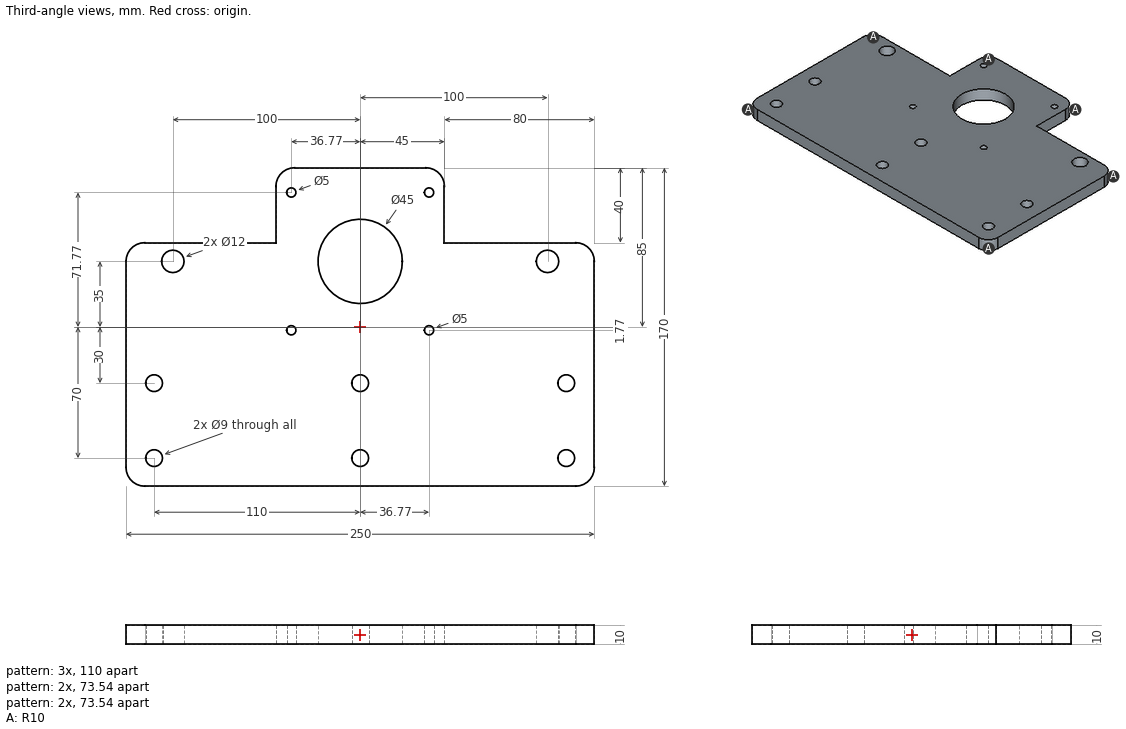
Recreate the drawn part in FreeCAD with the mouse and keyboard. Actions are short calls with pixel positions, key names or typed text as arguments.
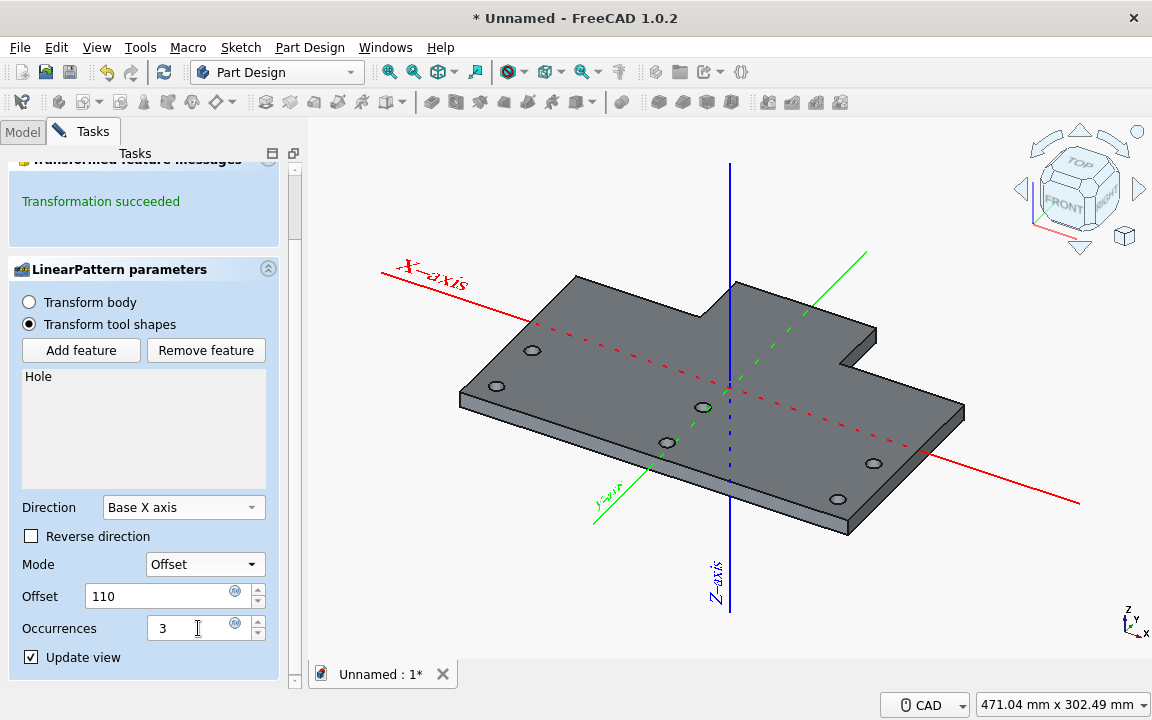
scroll(295, 426, up, 3)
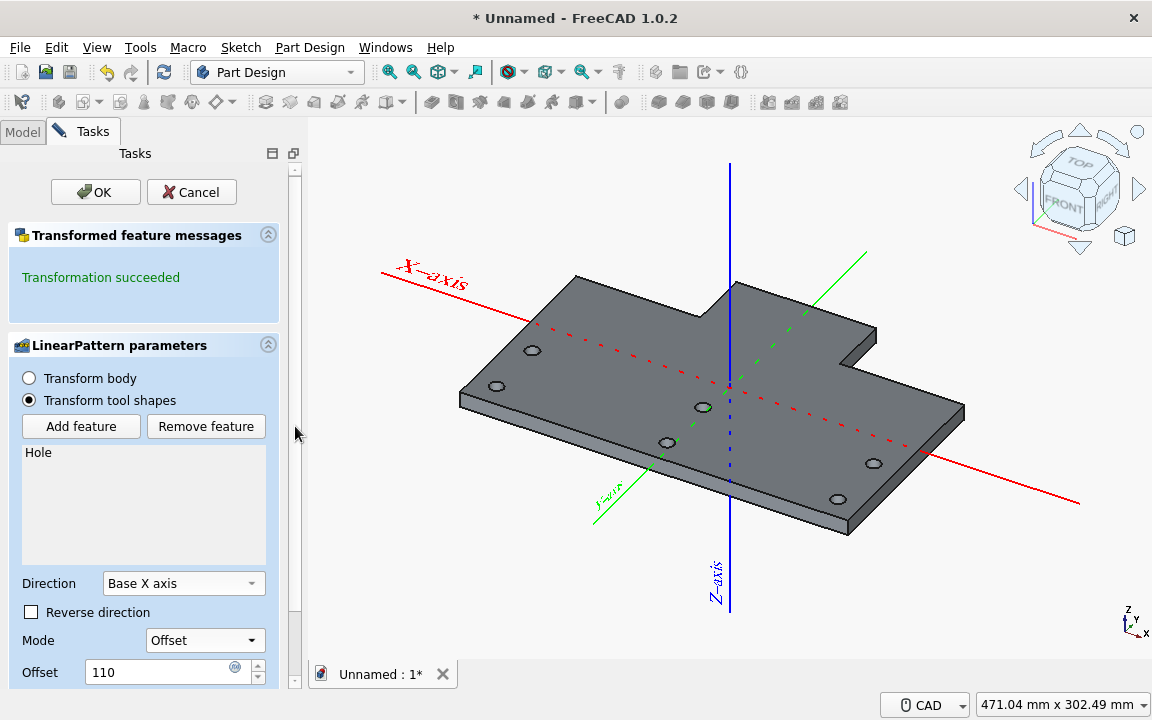
click(96, 192)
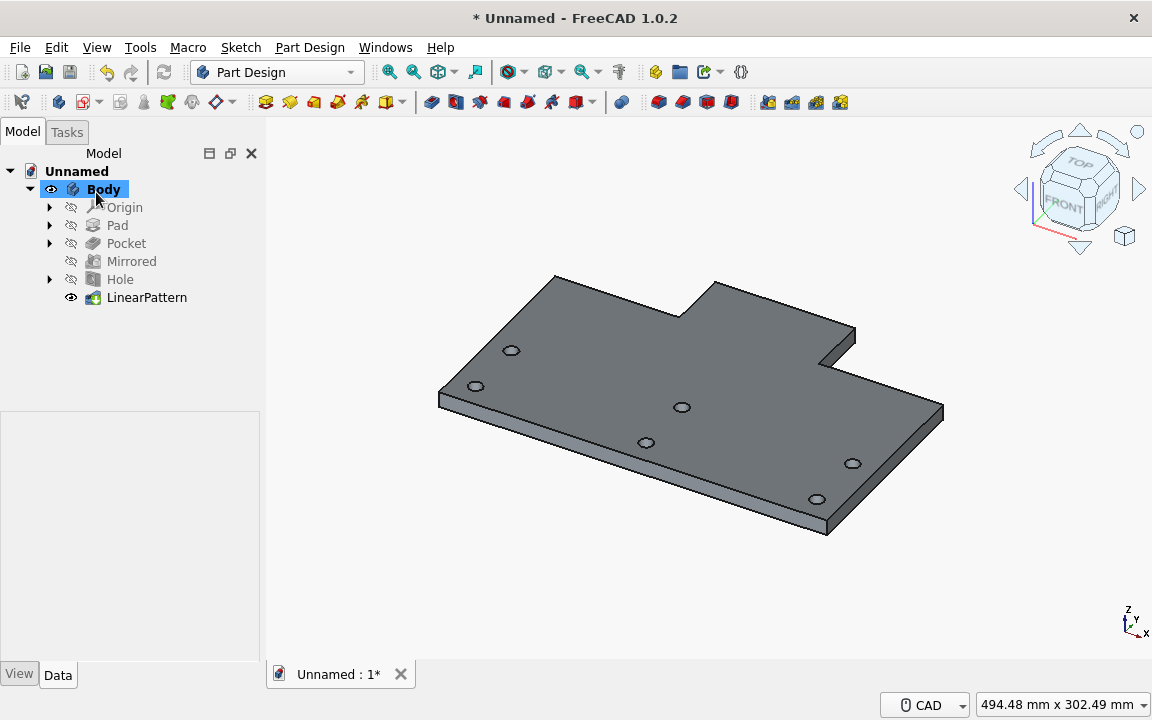
click(731, 358)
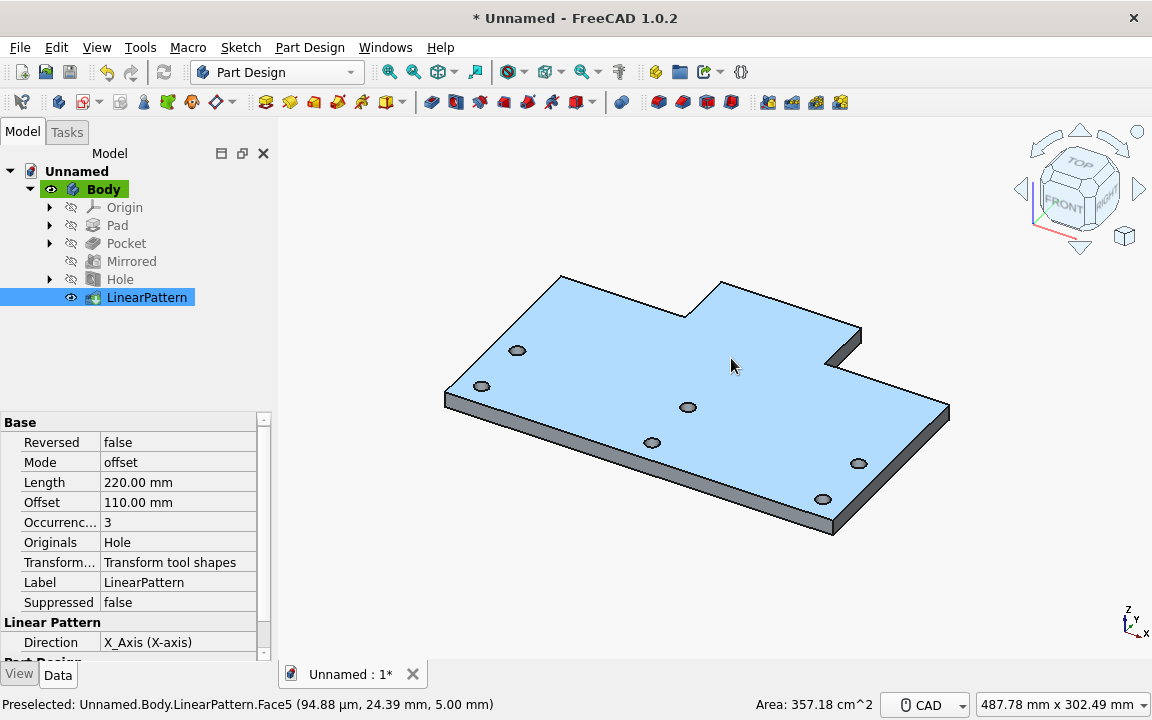
click(84, 102)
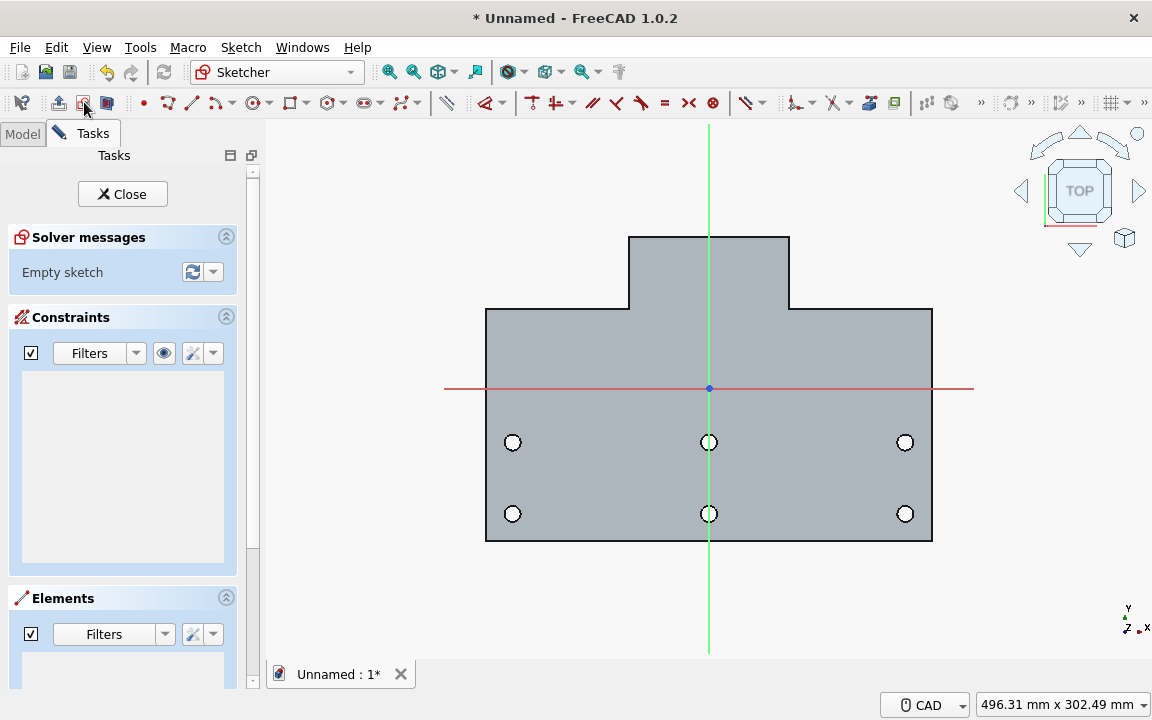
click(254, 104)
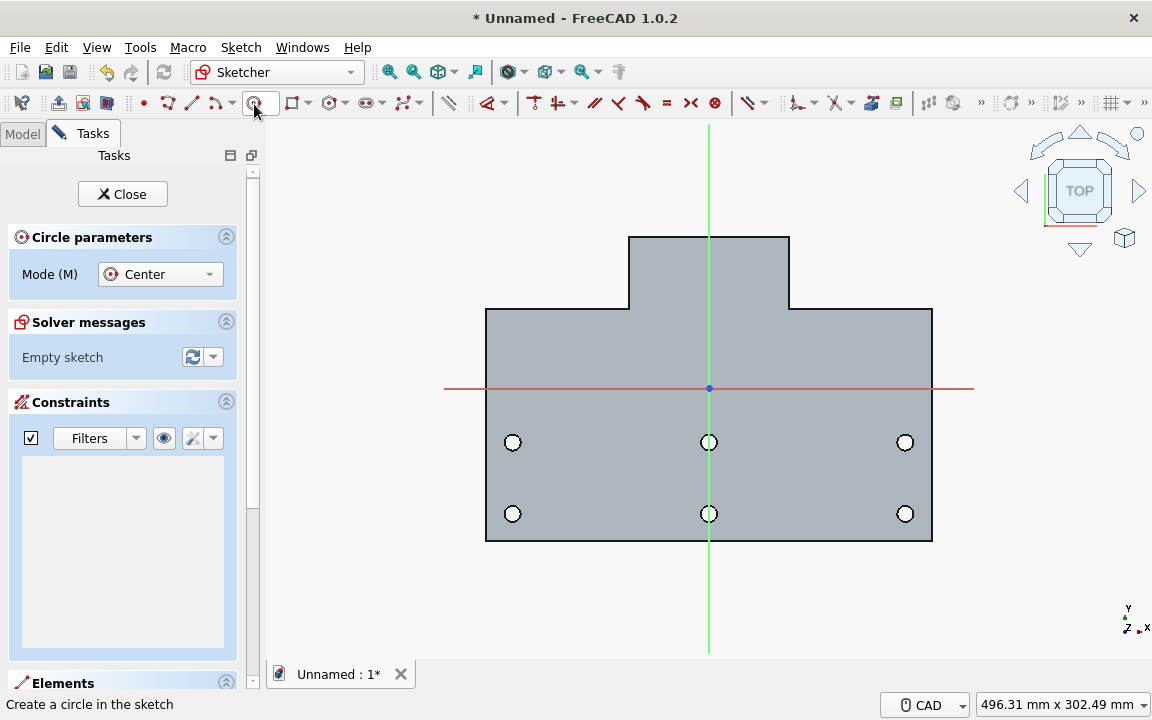
scroll(530, 327, up, 4)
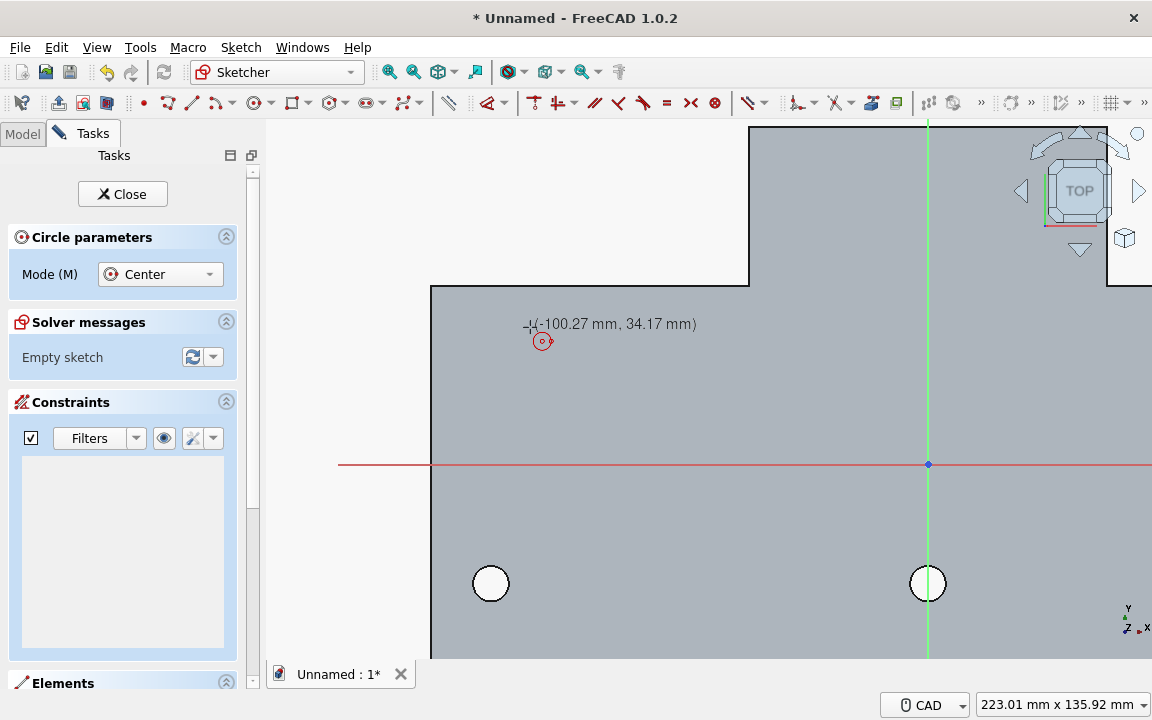
click(531, 325)
move(548, 309)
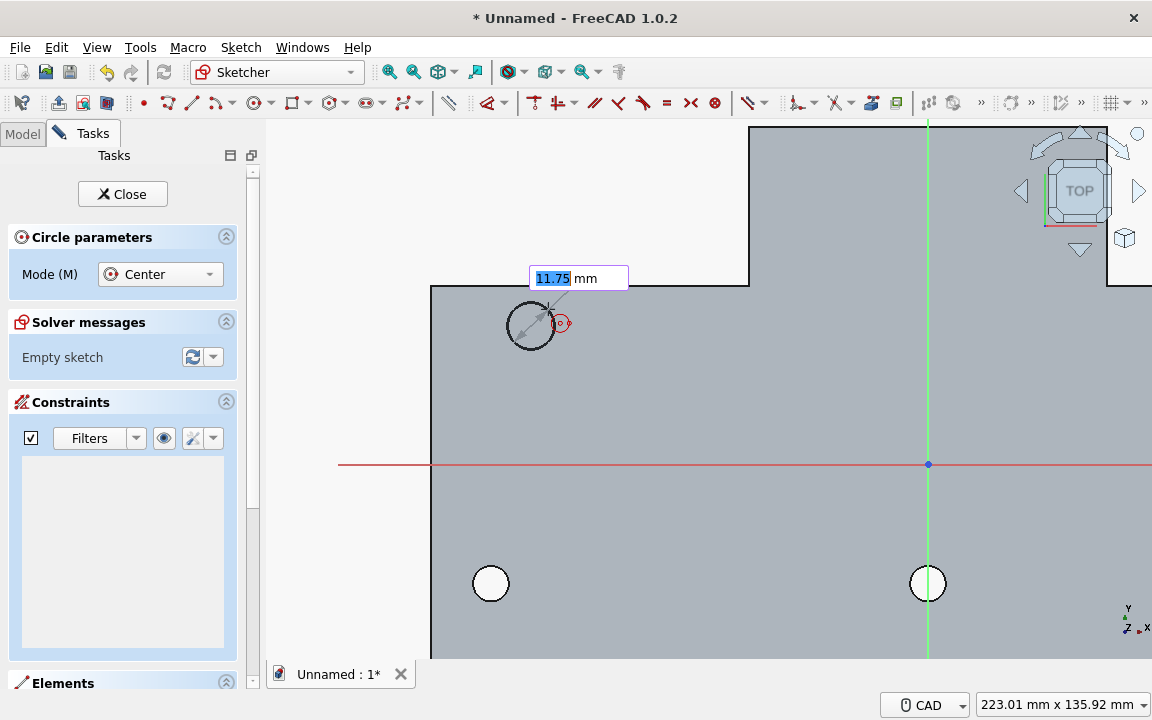
text(12)
key(Return)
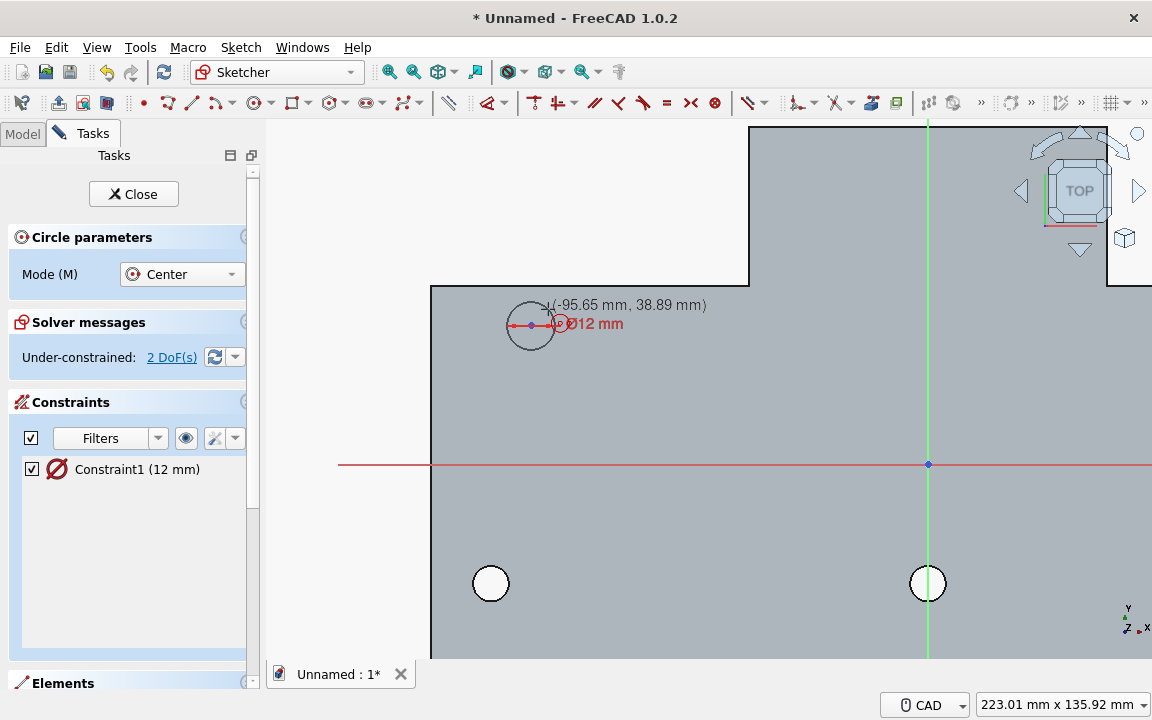
scroll(294, 396, down, 3)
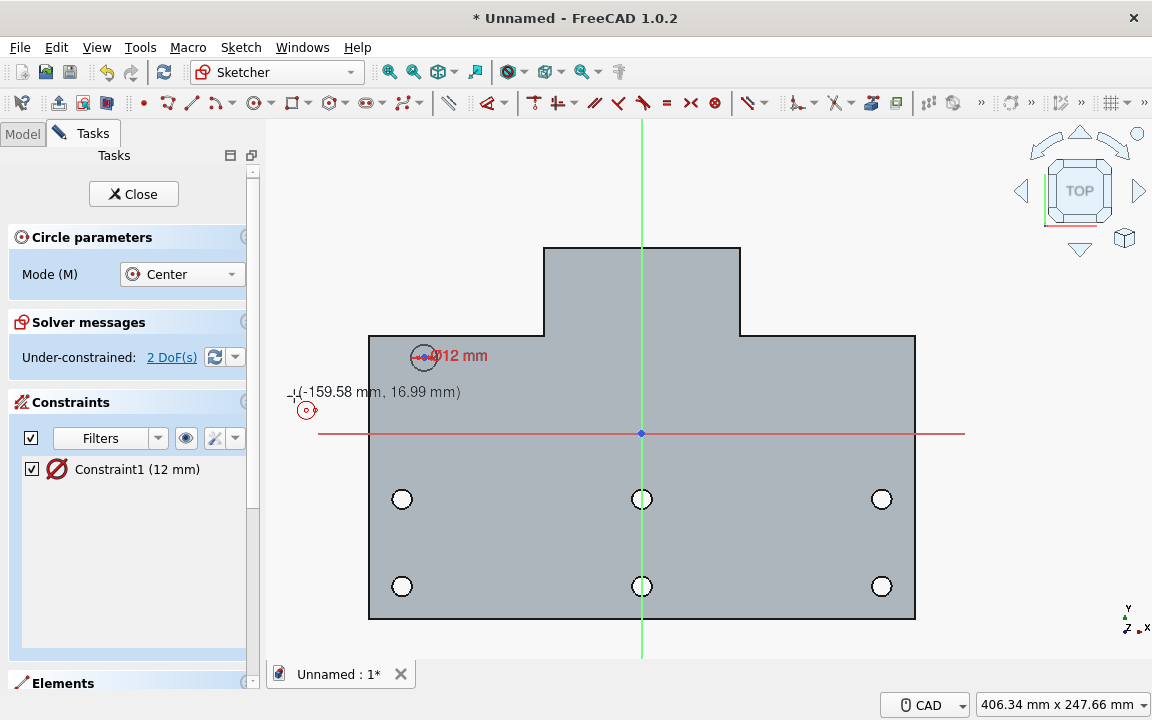
scroll(860, 358, up, 3)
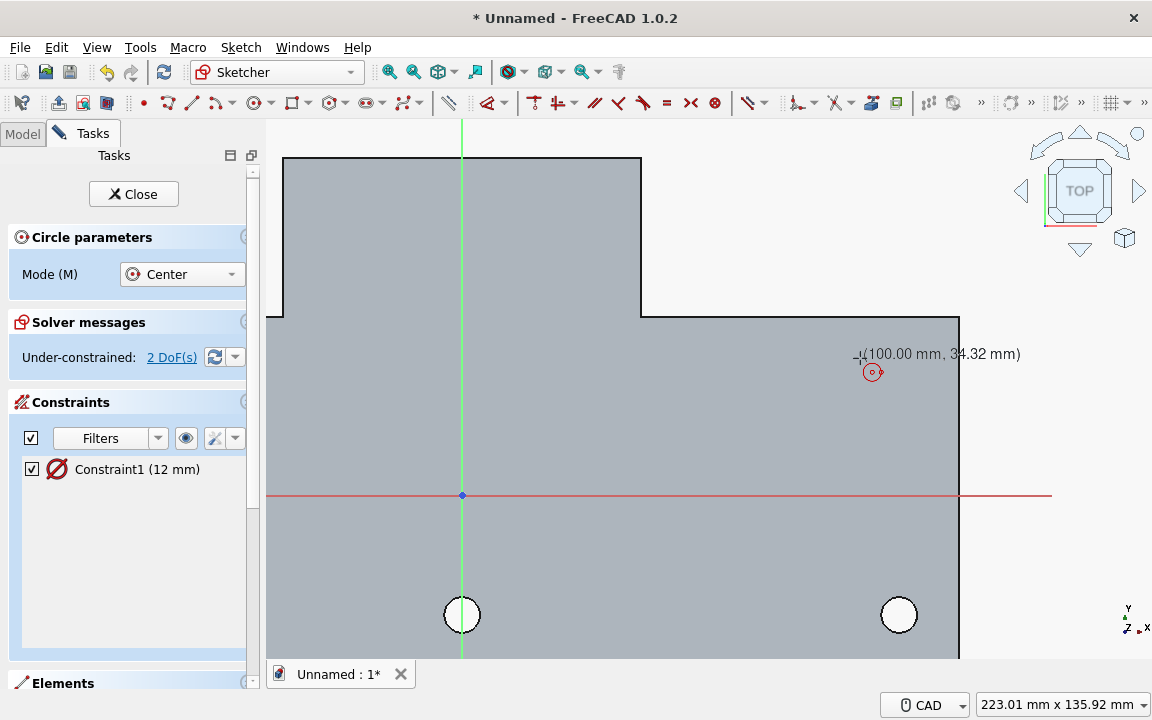
click(859, 357)
move(876, 340)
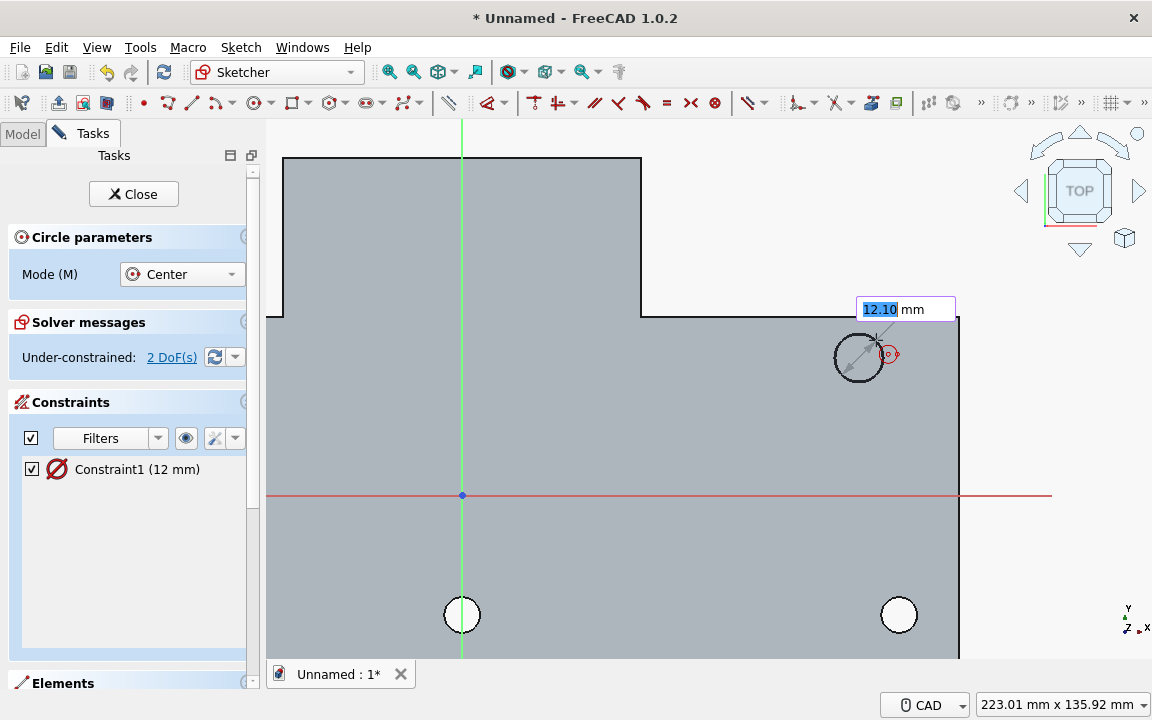
text(12)
key(Return)
key(Escape)